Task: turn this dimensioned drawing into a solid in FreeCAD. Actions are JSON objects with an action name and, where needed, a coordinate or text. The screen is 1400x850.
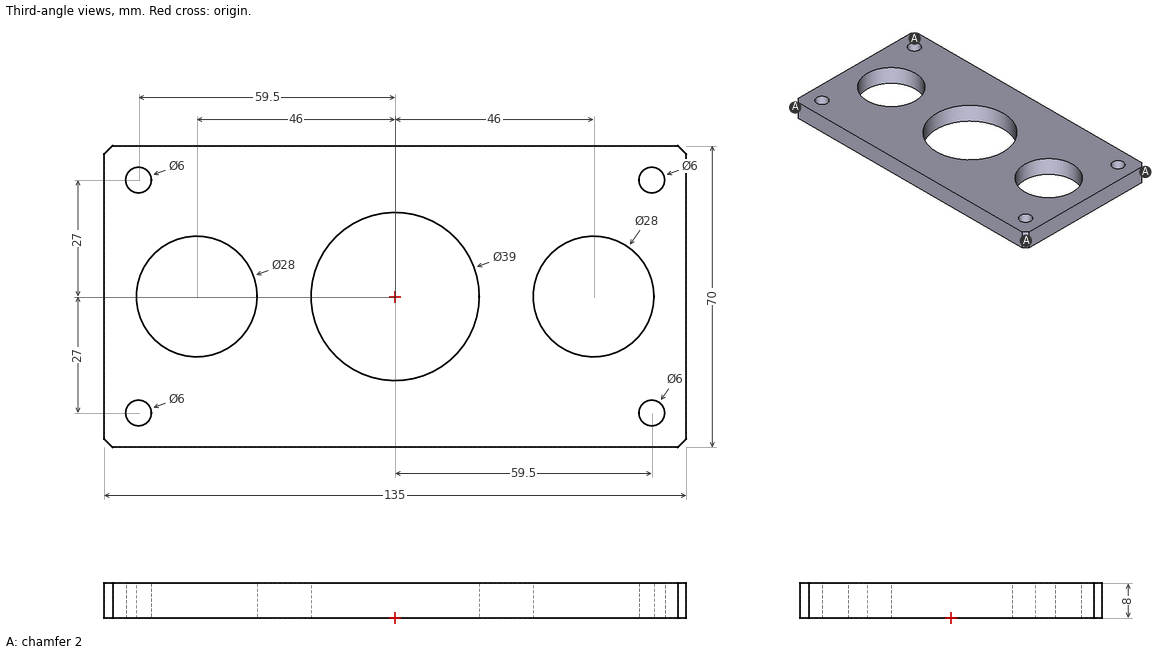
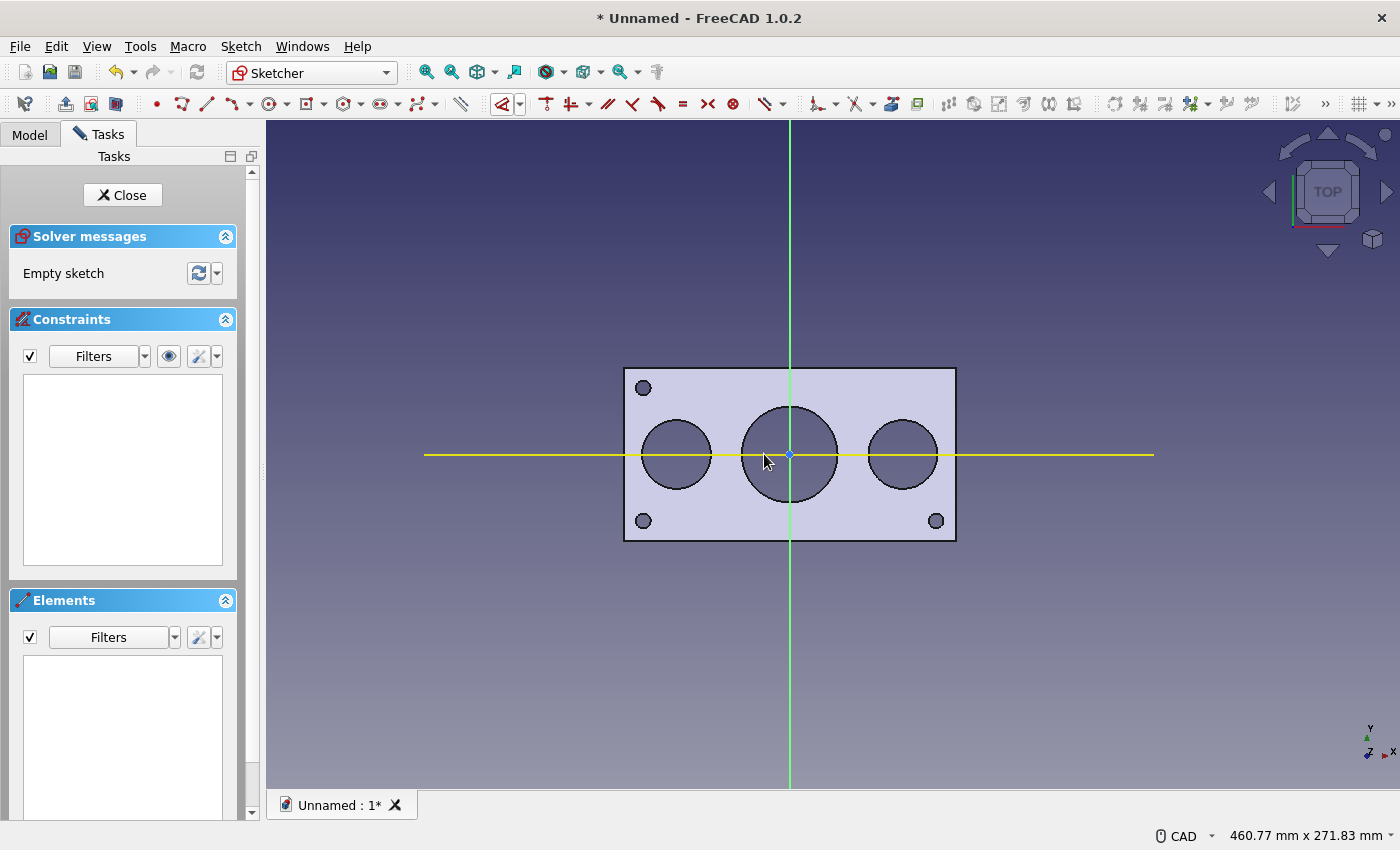
{"action": "scroll", "coordinate": [945, 385], "scroll_direction": "up", "scroll_amount": 15}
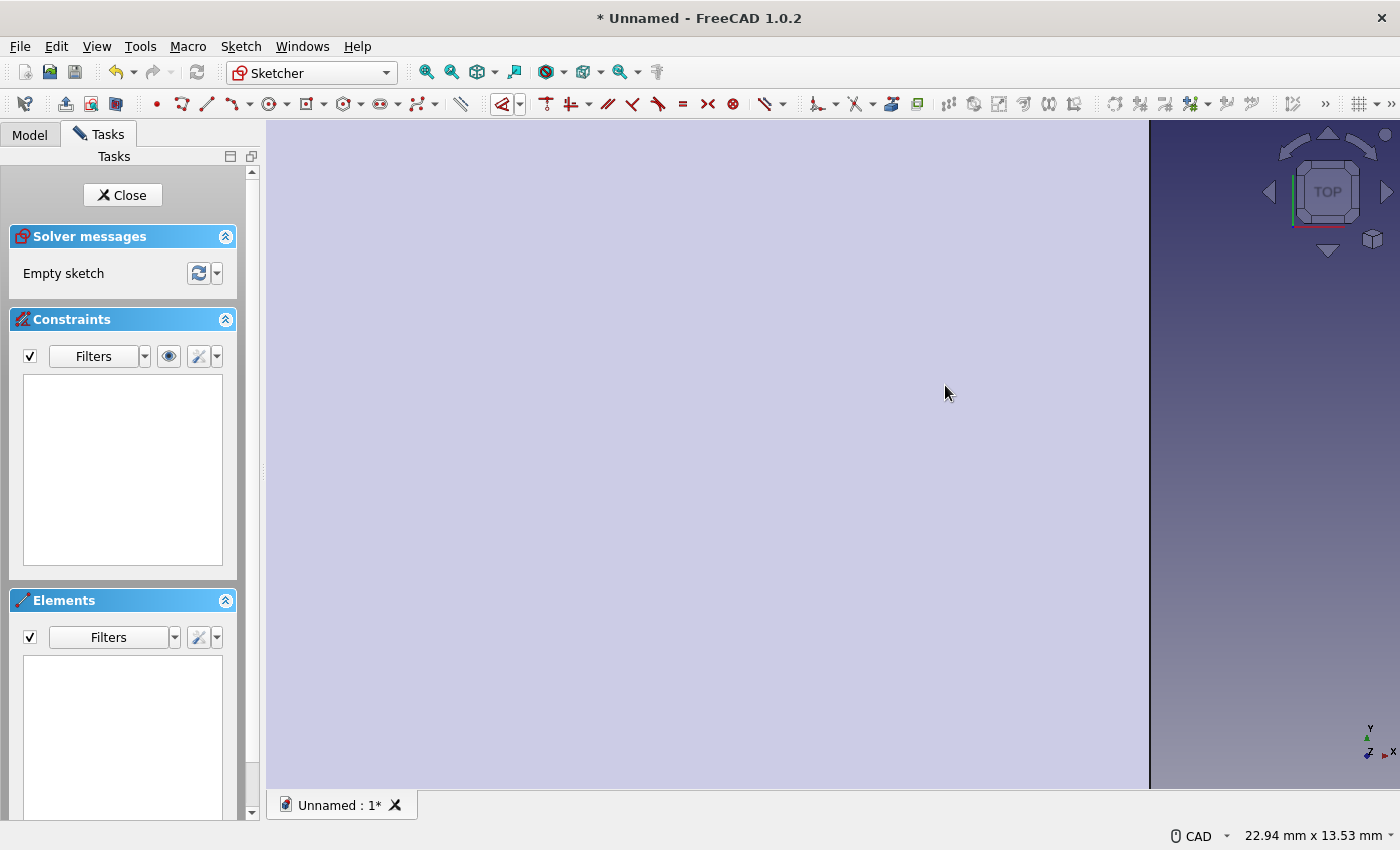
{"action": "scroll", "coordinate": [735, 407], "scroll_direction": "up", "scroll_amount": 2}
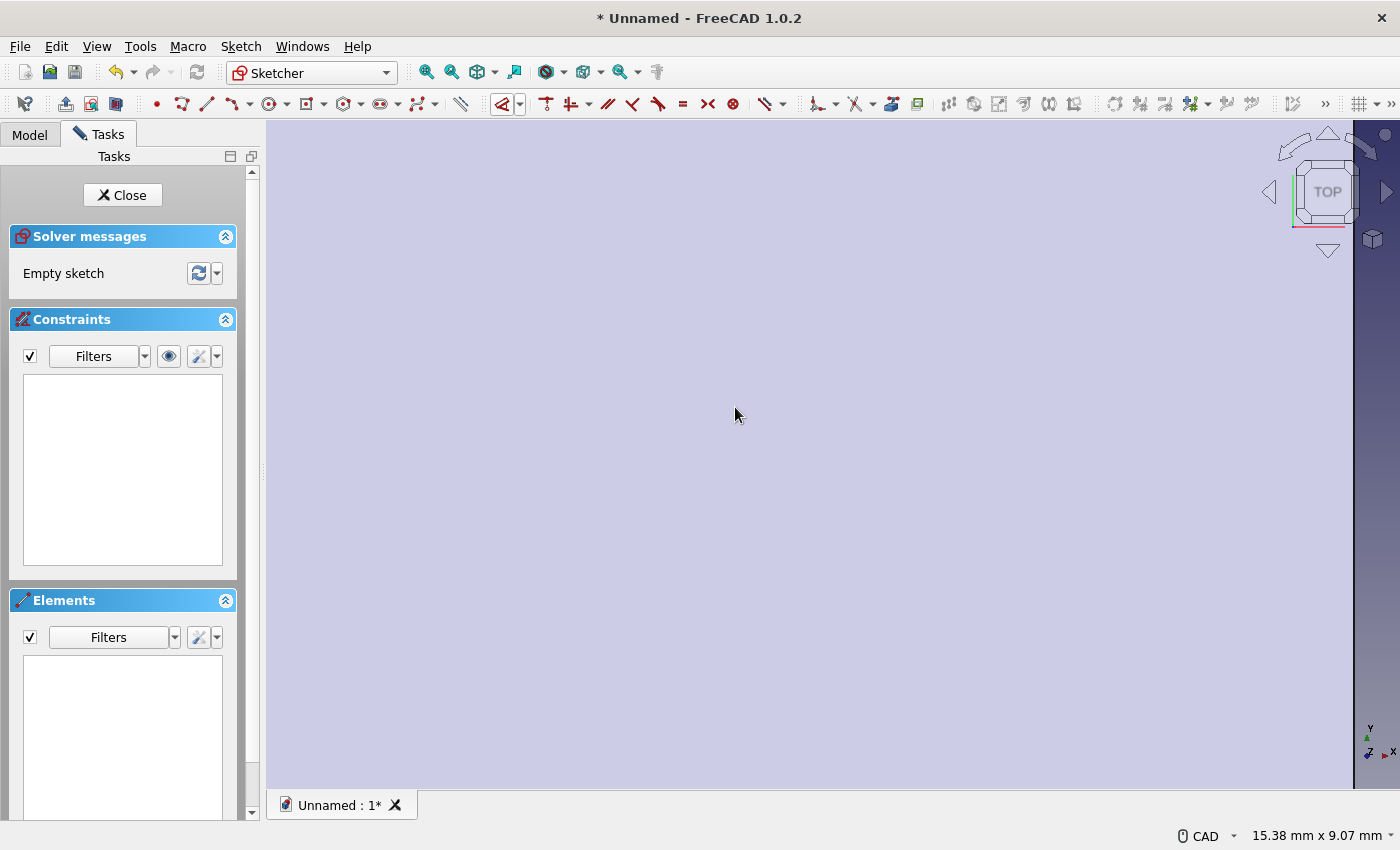
{"action": "key", "text": "g c"}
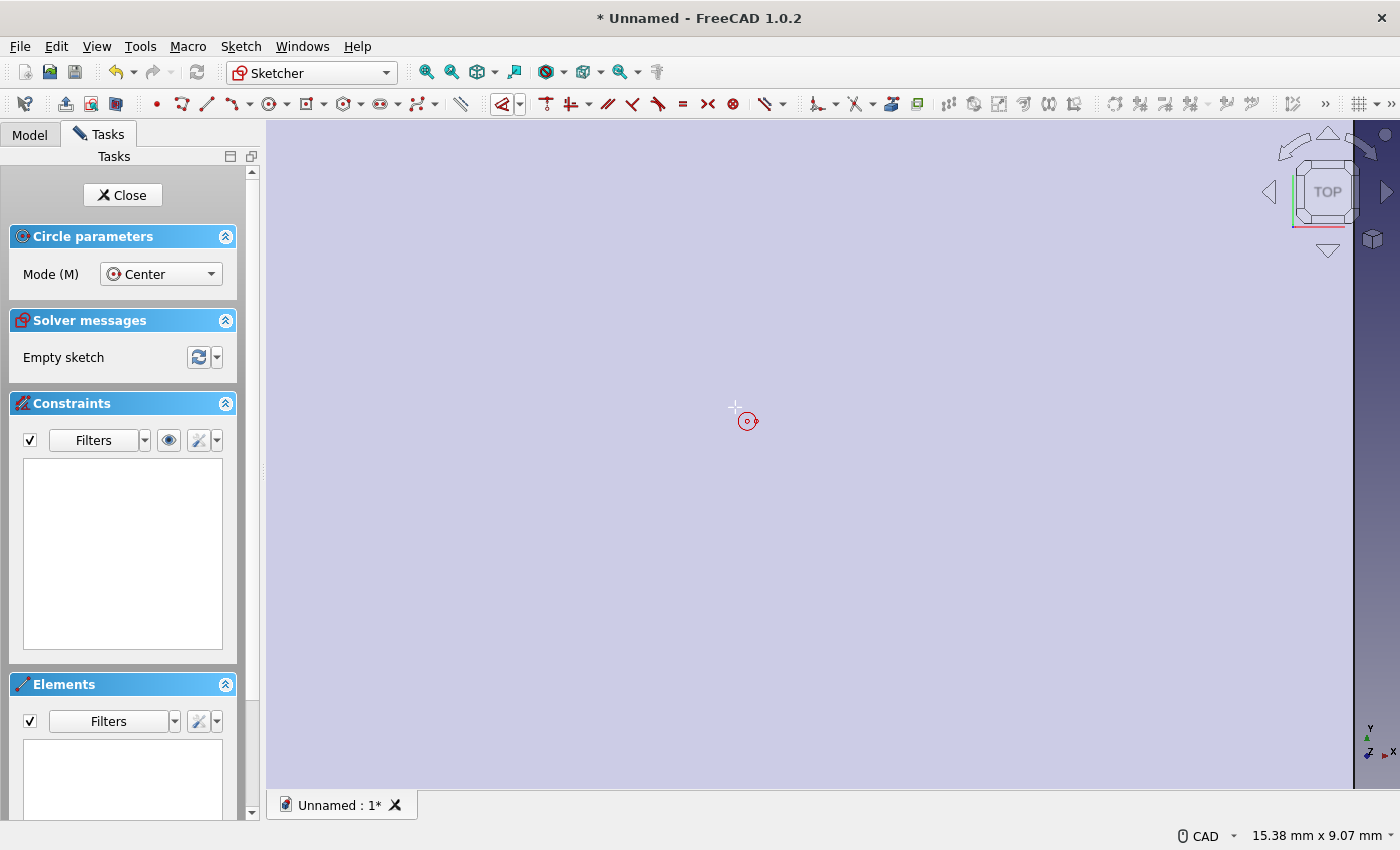
{"action": "left_click", "coordinate": [764, 454]}
{"action": "left_click", "coordinate": [921, 298]}
{"action": "key", "text": "Escape"}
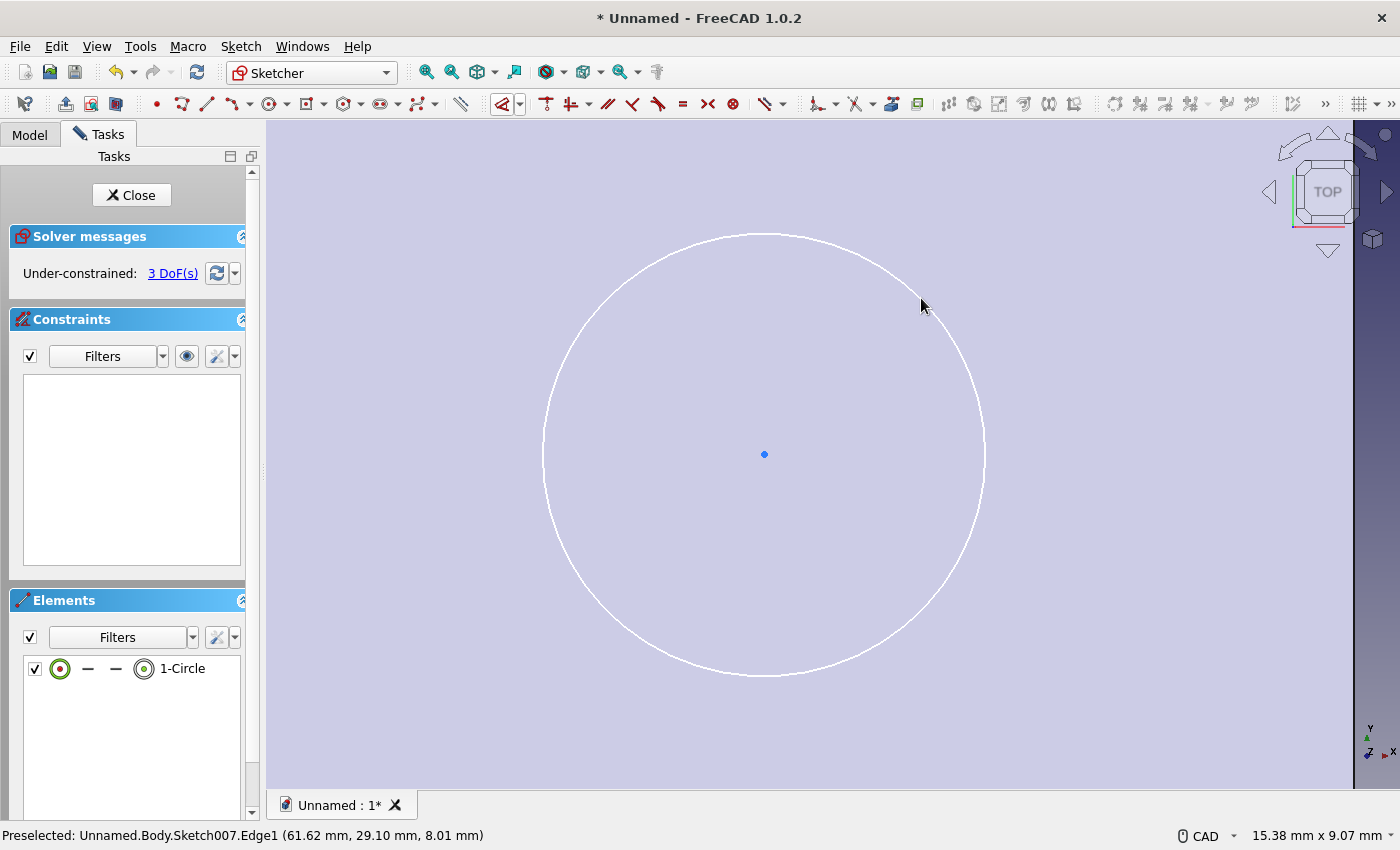
{"action": "left_click", "coordinate": [920, 298]}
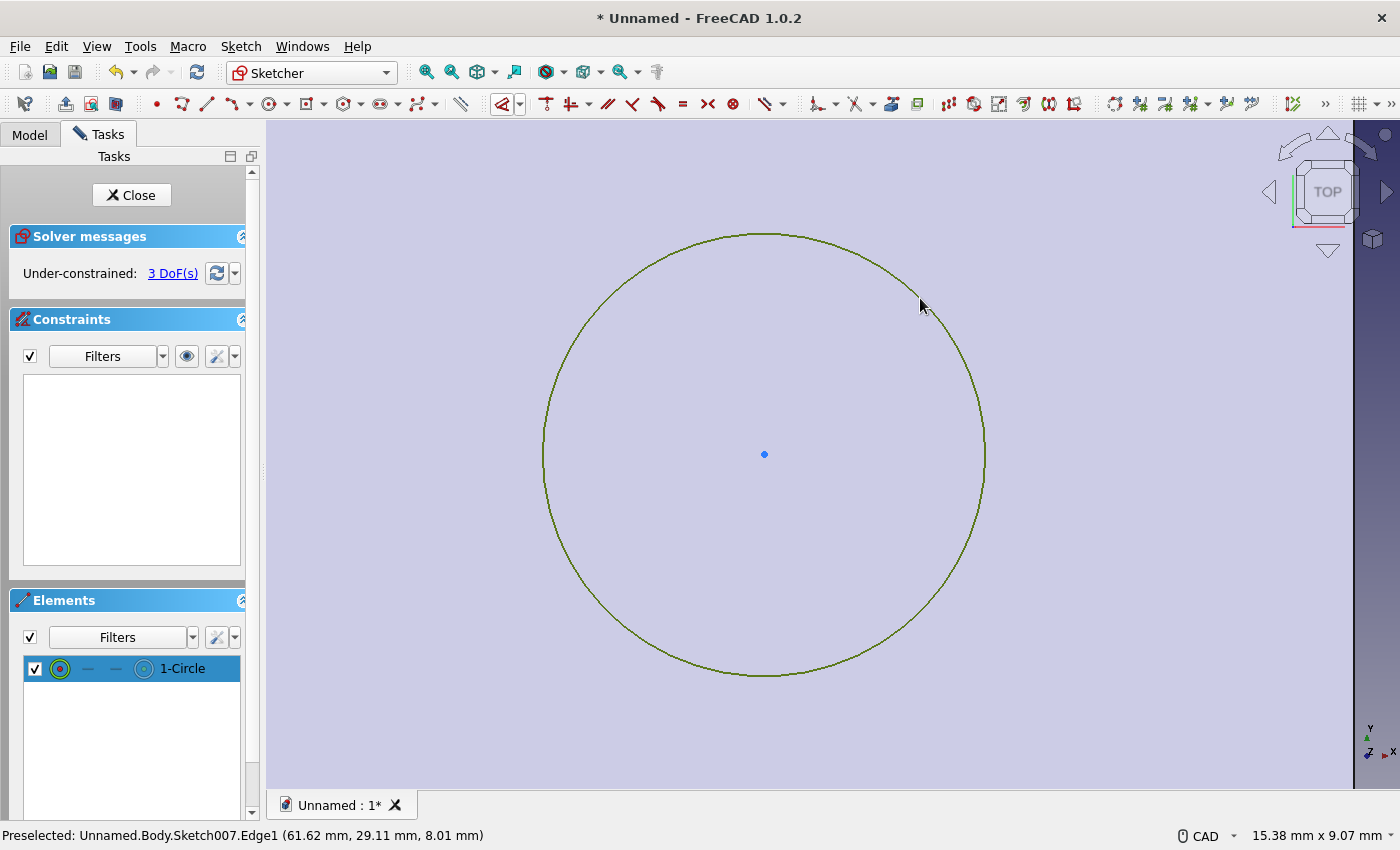
{"action": "key", "text": "k o"}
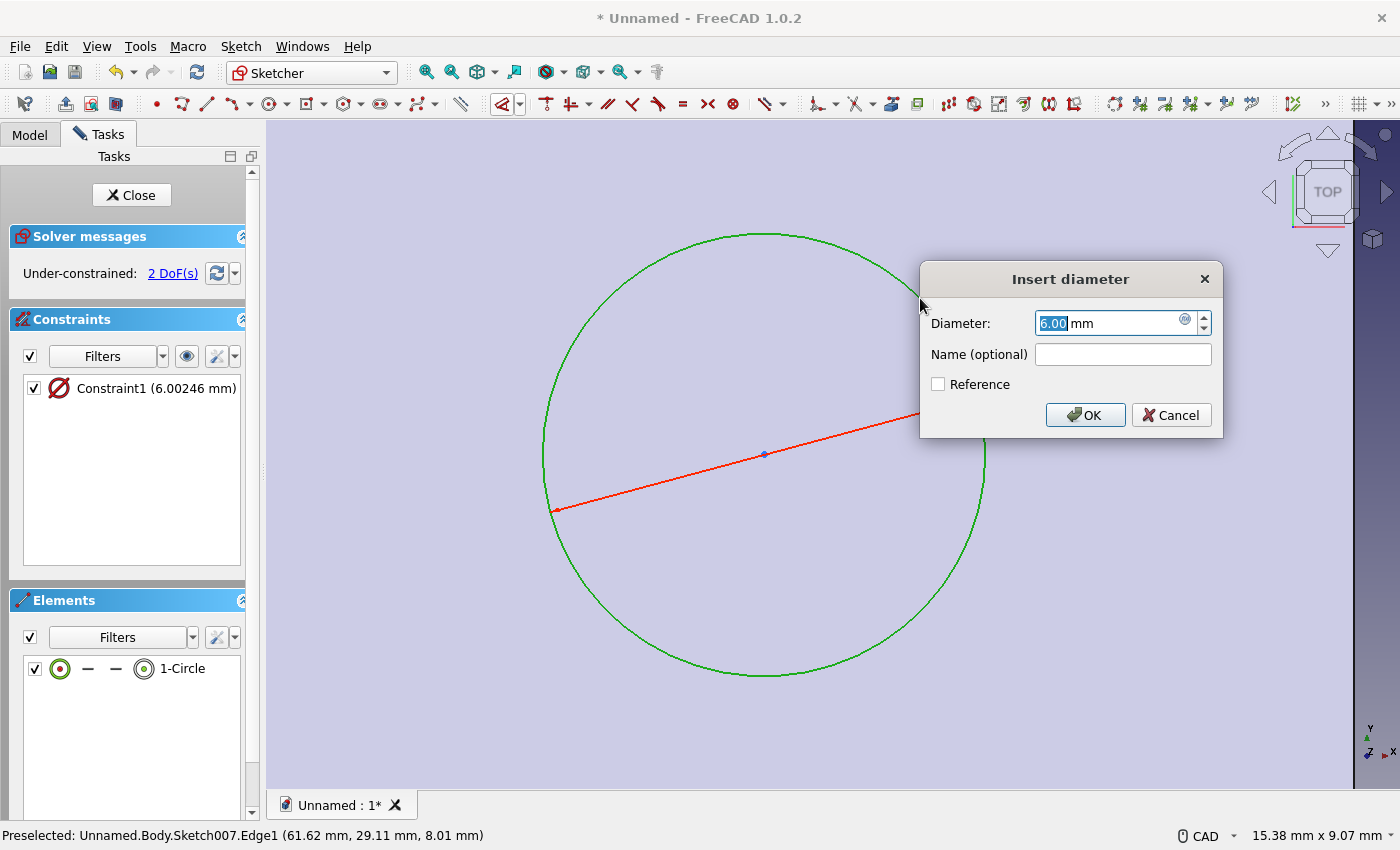
{"action": "type", "text": "6"}
{"action": "key", "text": "Return"}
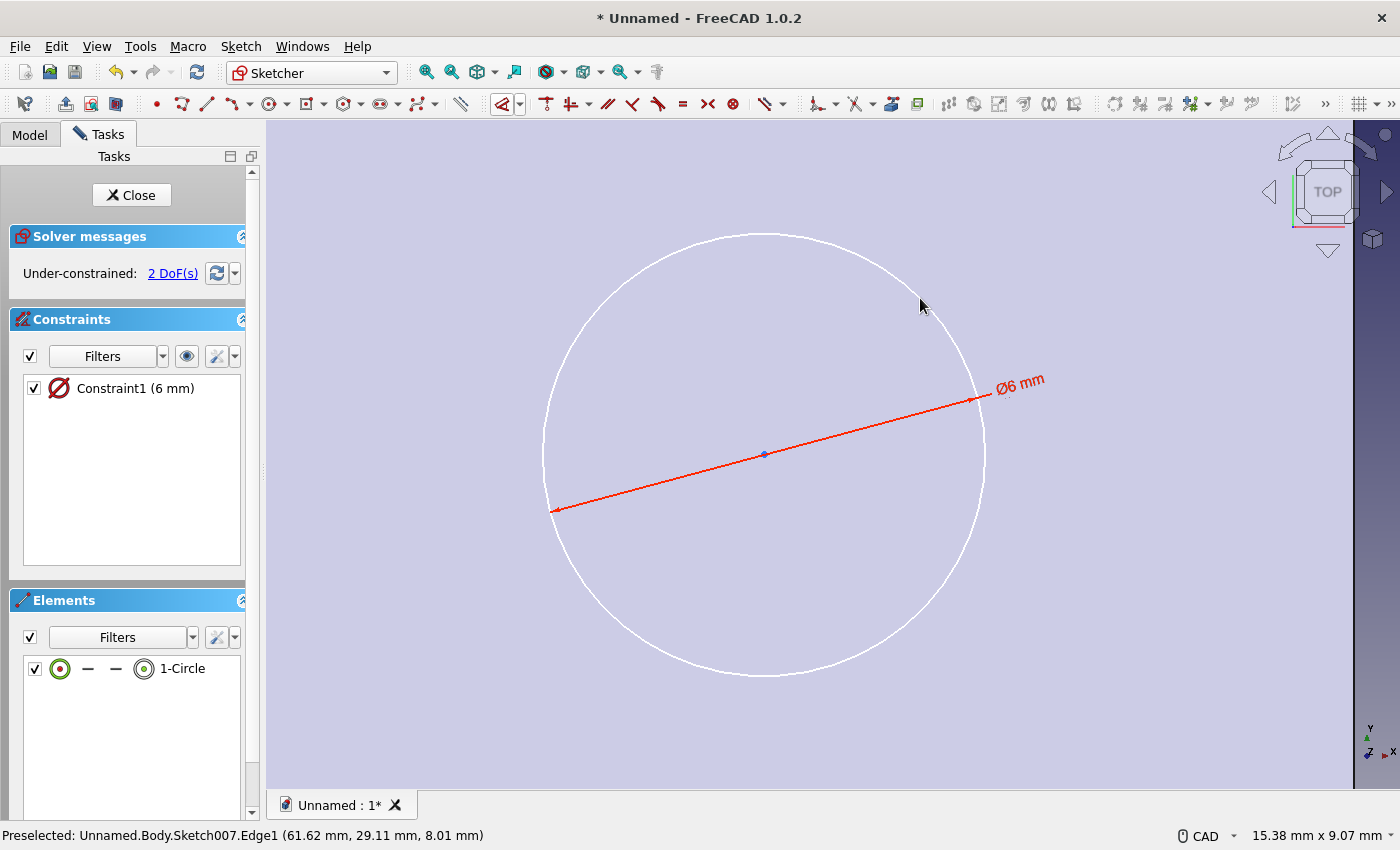
{"action": "left_click", "coordinate": [764, 455]}